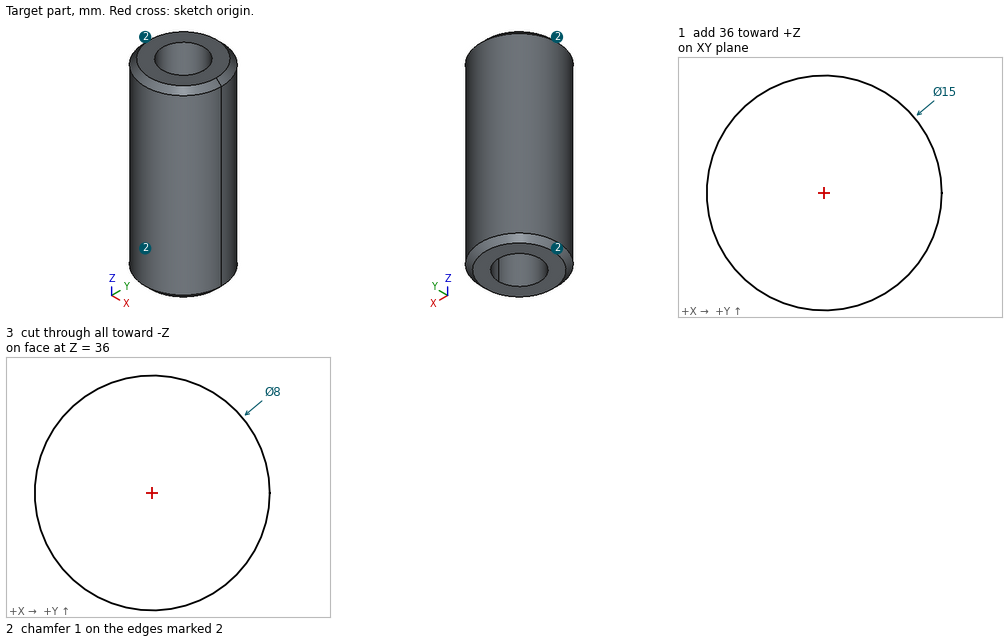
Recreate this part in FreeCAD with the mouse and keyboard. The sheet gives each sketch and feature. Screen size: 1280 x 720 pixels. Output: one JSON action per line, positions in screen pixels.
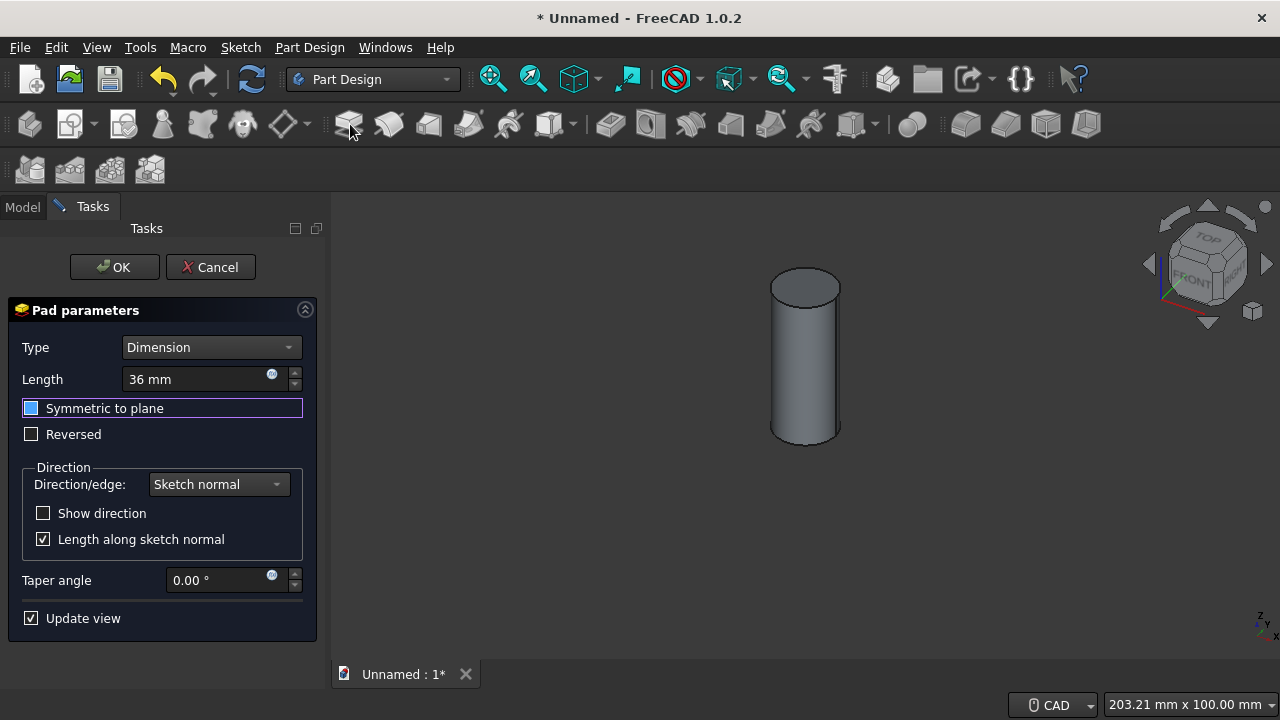
{"action": "left_click", "coordinate": [115, 267]}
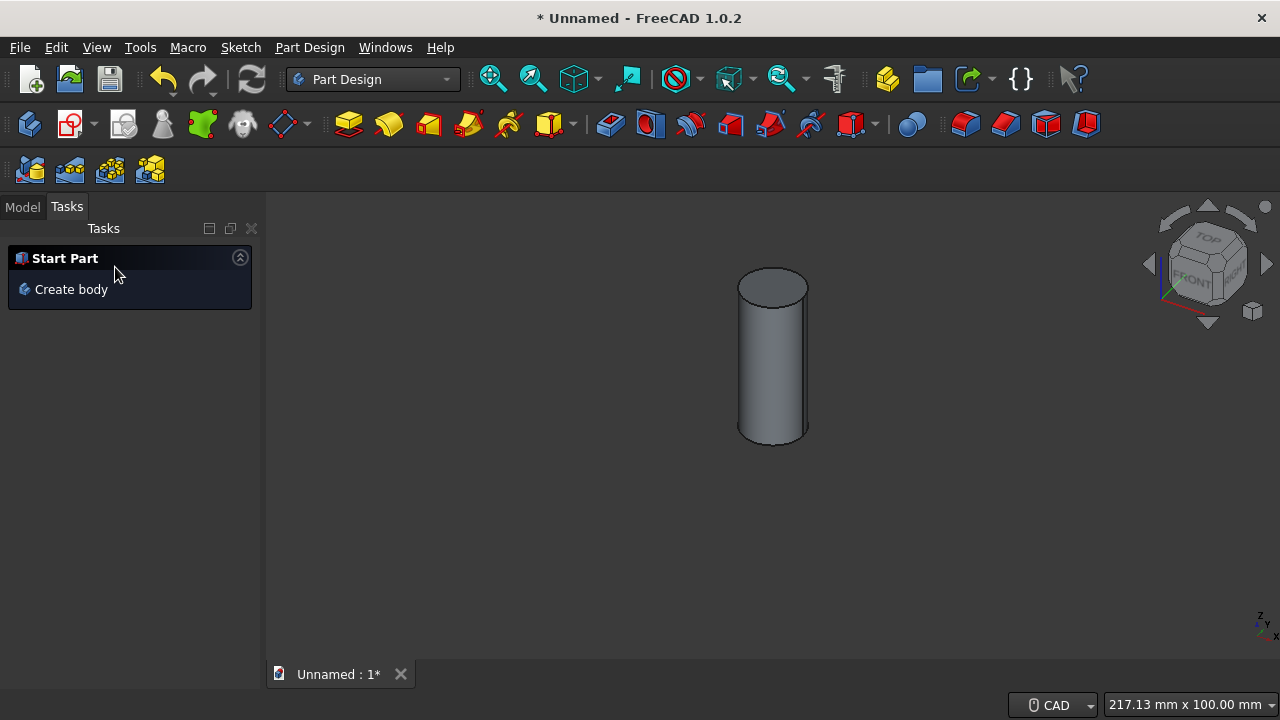
{"action": "left_click", "coordinate": [494, 80]}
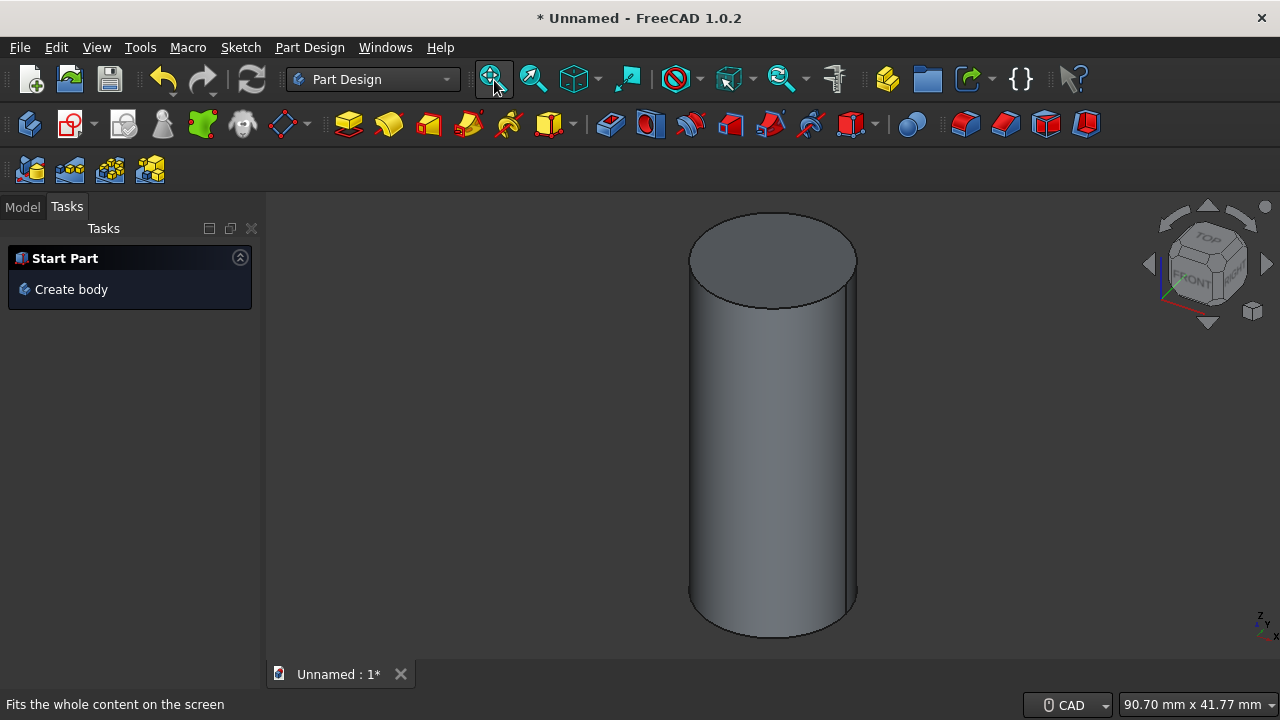
{"action": "left_click", "coordinate": [690, 265]}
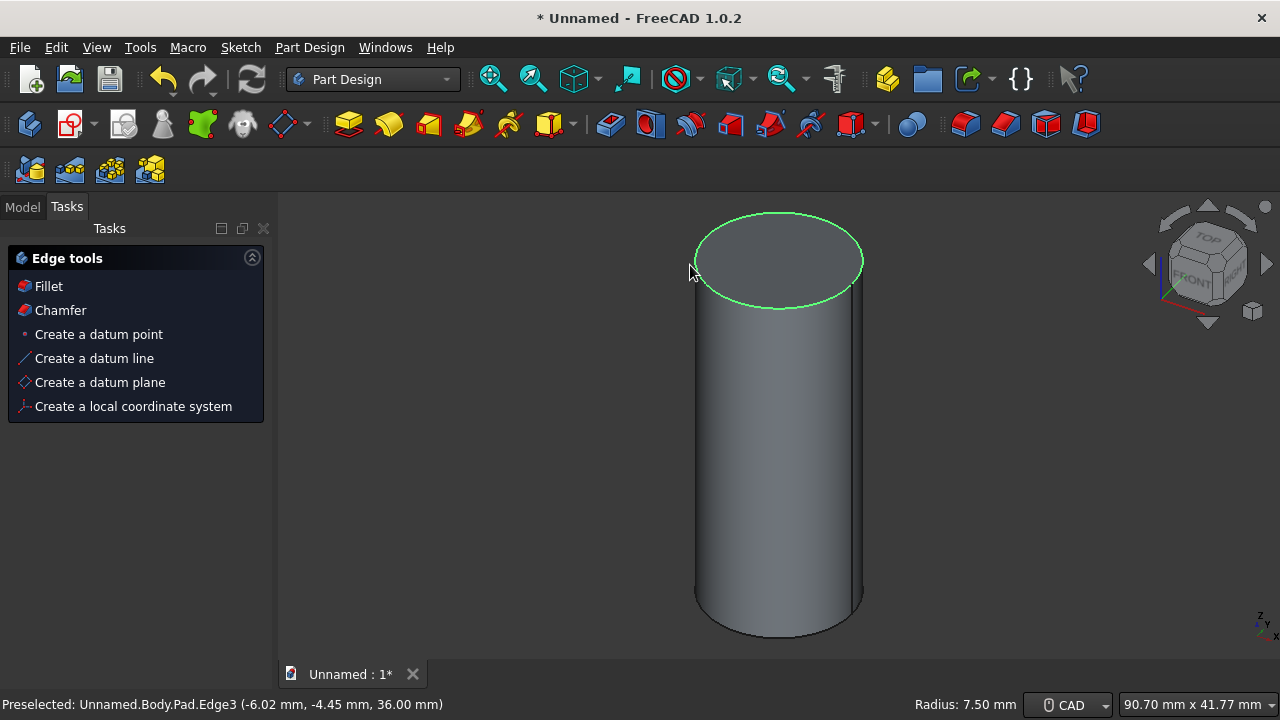
{"action": "key", "text": "0"}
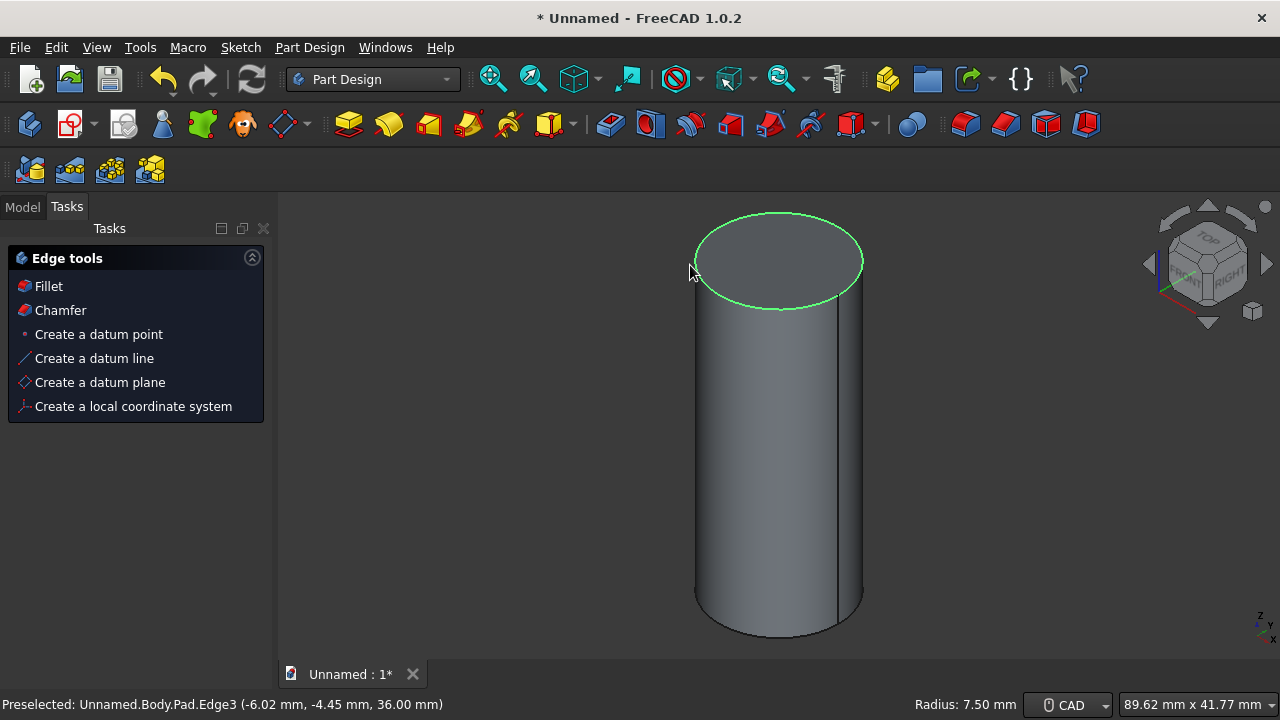
{"action": "key", "text": "2"}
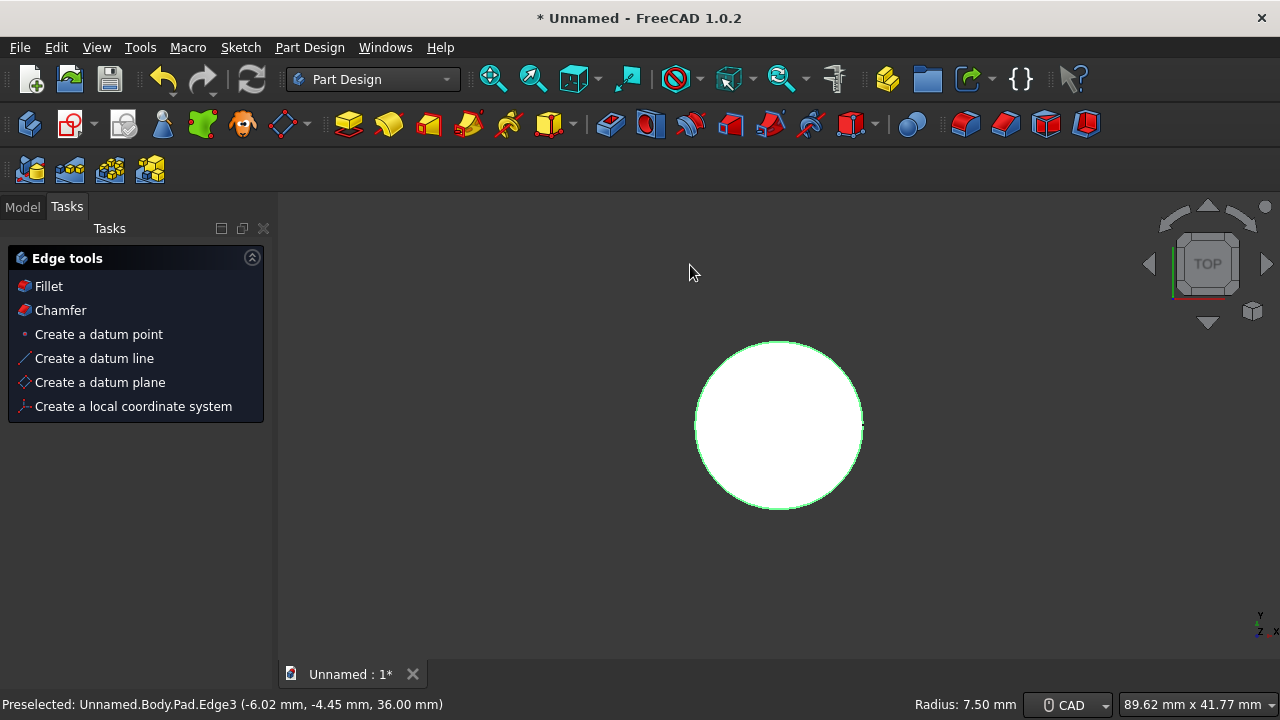
{"action": "left_click", "coordinate": [494, 80]}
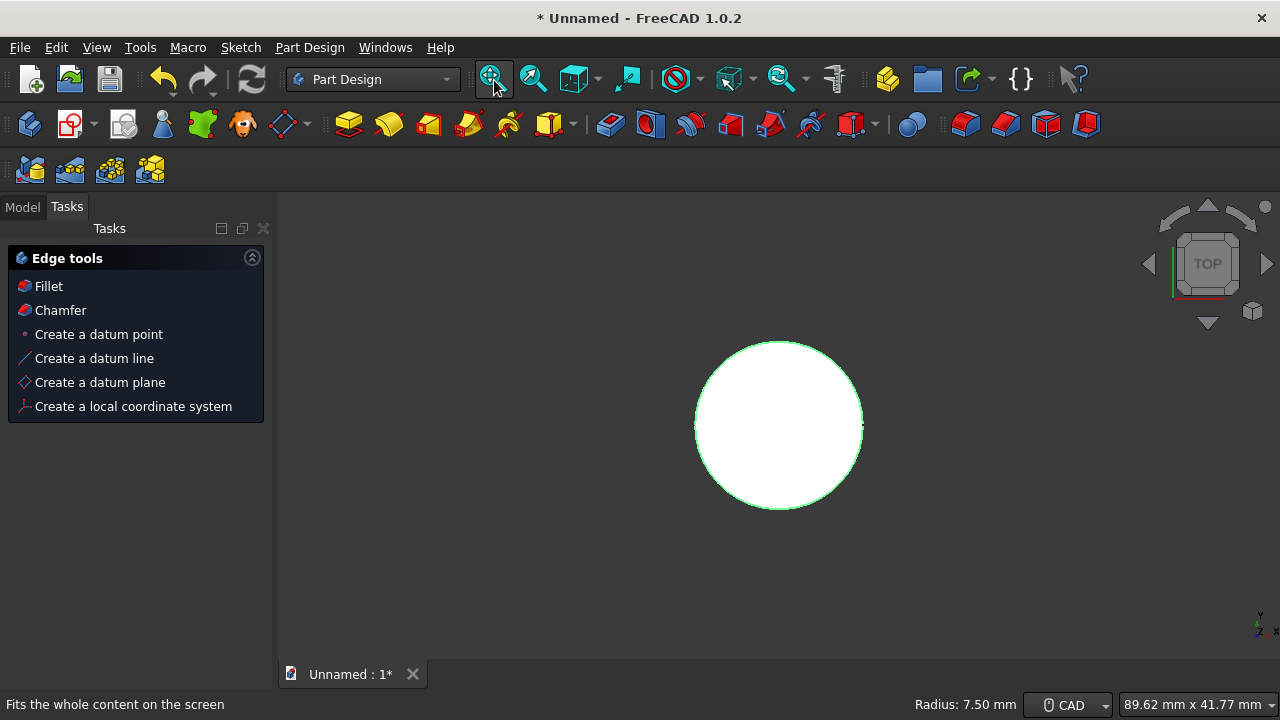
{"action": "key", "text": "1"}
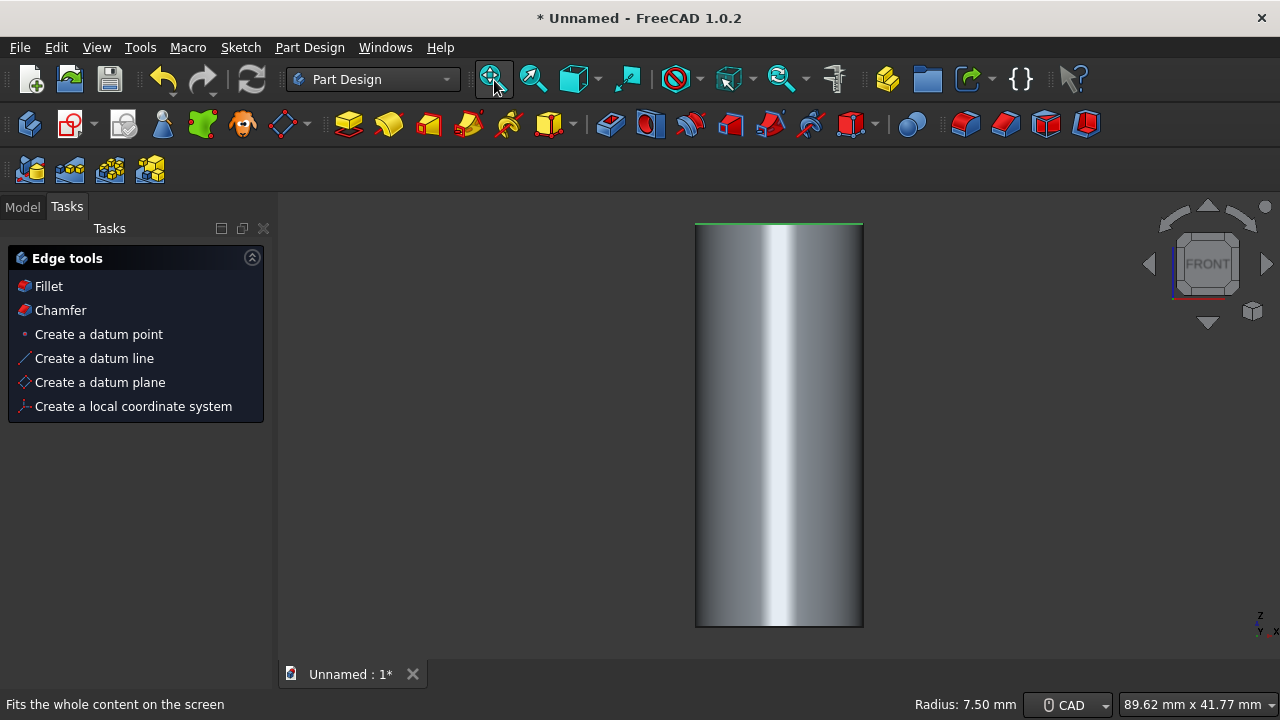
{"action": "left_click", "coordinate": [711, 626], "text": "ctrl"}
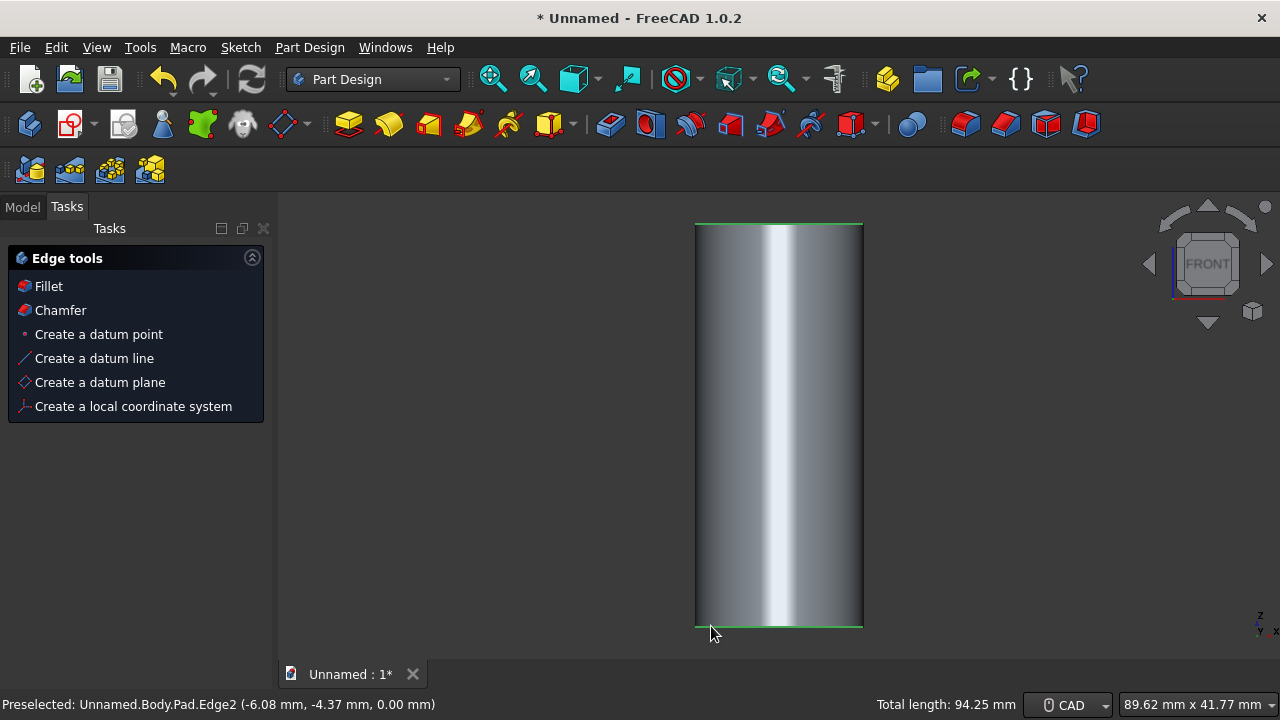
{"action": "left_click", "coordinate": [1006, 124]}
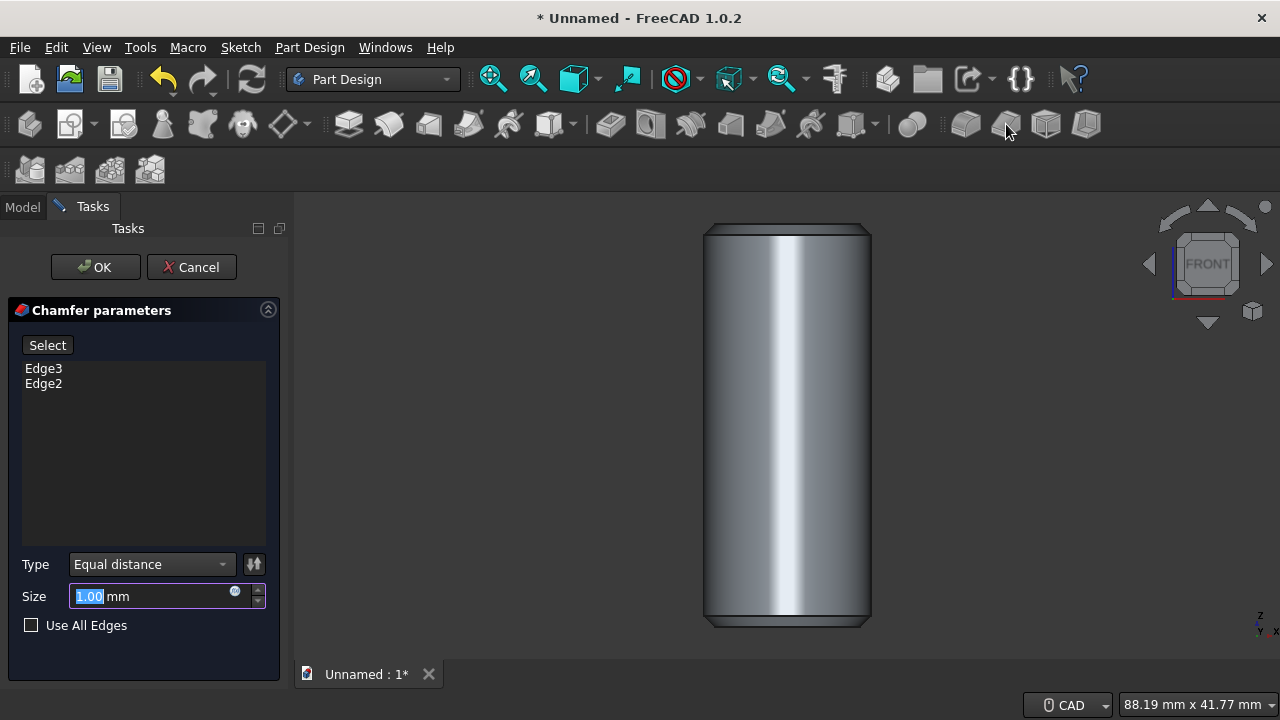
{"action": "type", "text": "1"}
{"action": "key", "text": "Tab"}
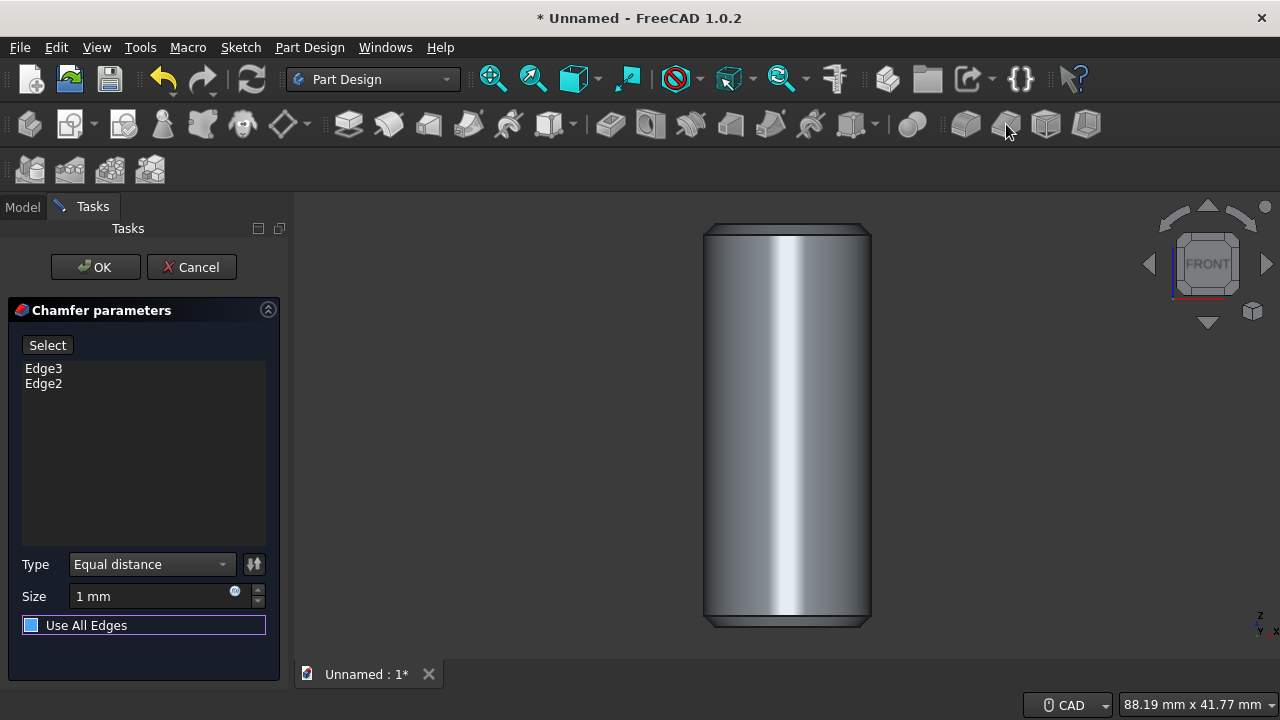
{"action": "left_click", "coordinate": [96, 267]}